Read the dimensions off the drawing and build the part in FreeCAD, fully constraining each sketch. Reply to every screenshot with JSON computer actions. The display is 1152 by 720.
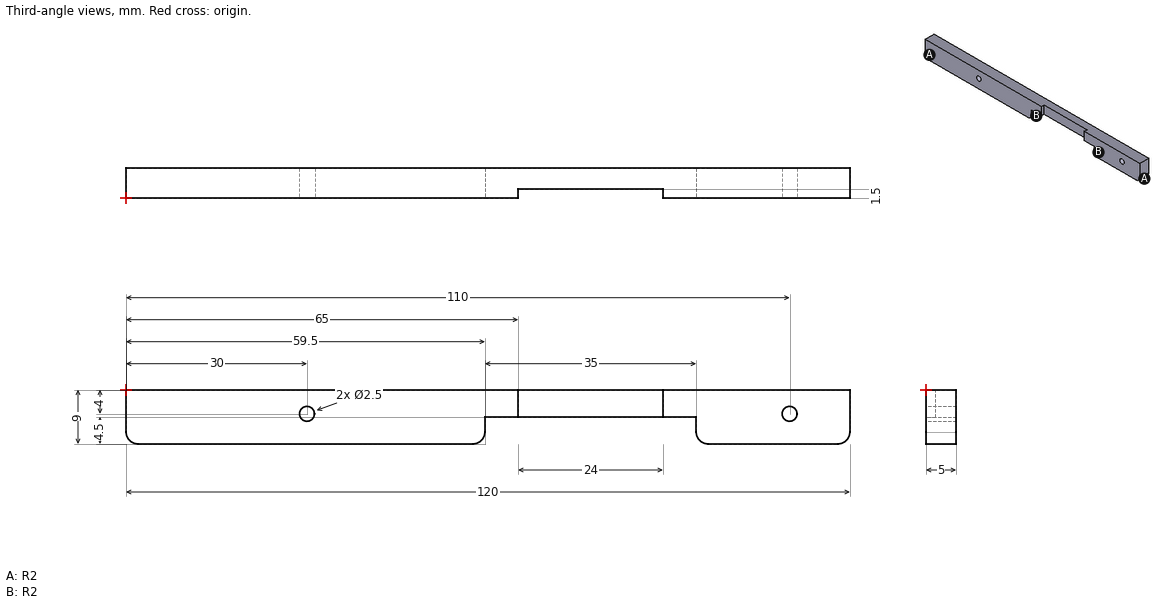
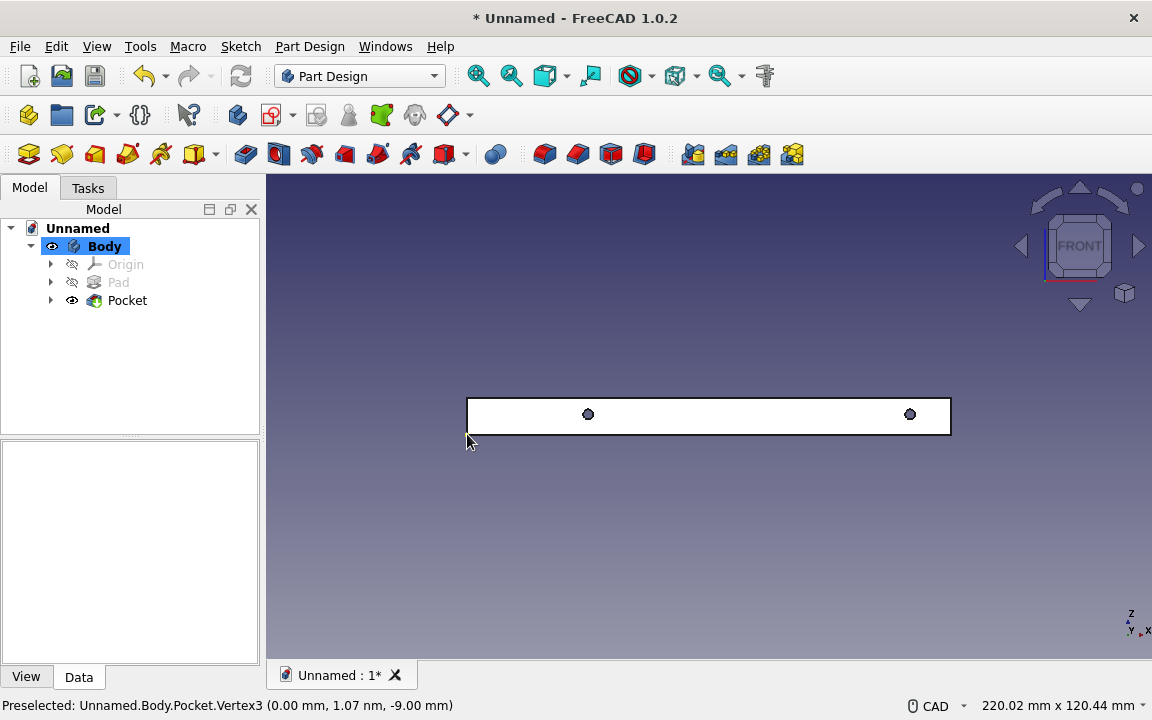
{"action": "key", "text": "3"}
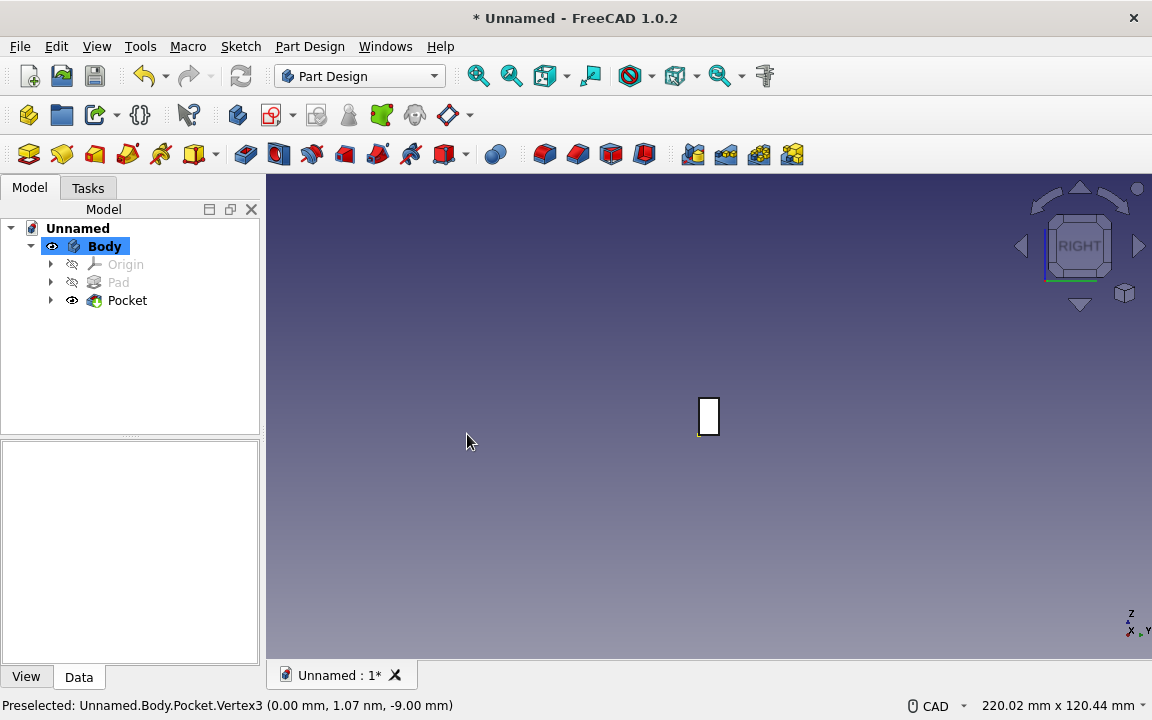
{"action": "key", "text": "v f"}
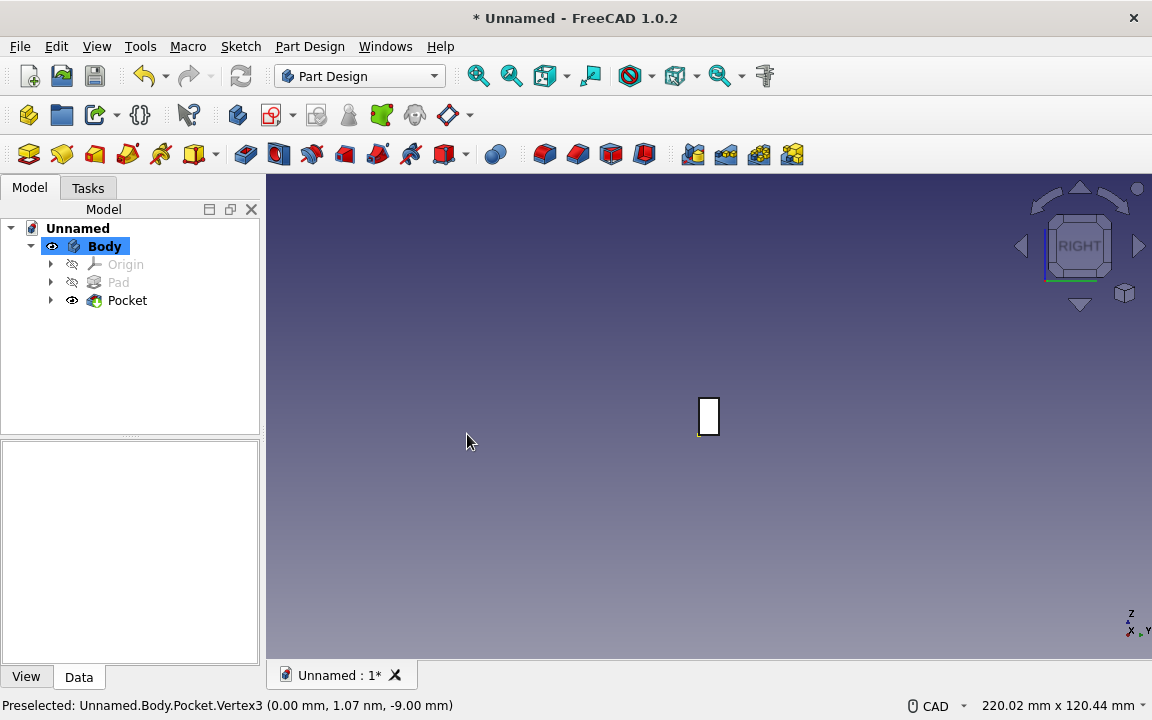
{"action": "left_click", "coordinate": [709, 434]}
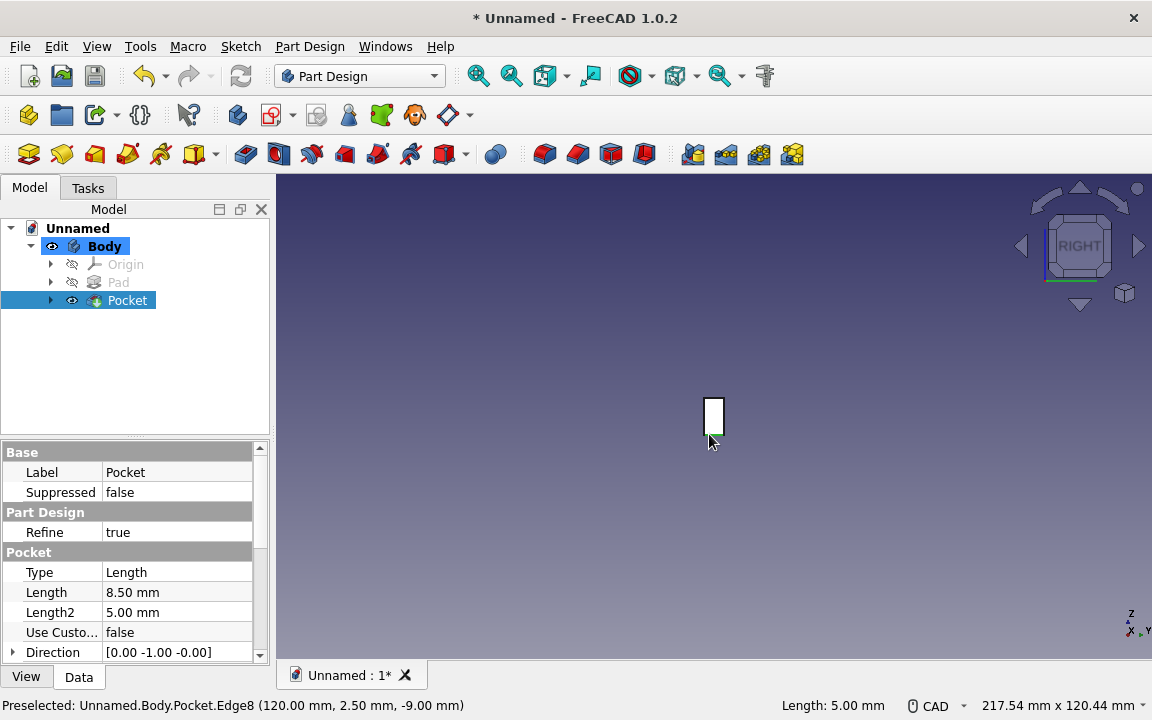
{"action": "scroll", "coordinate": [714, 434], "scroll_direction": "up", "scroll_amount": 4}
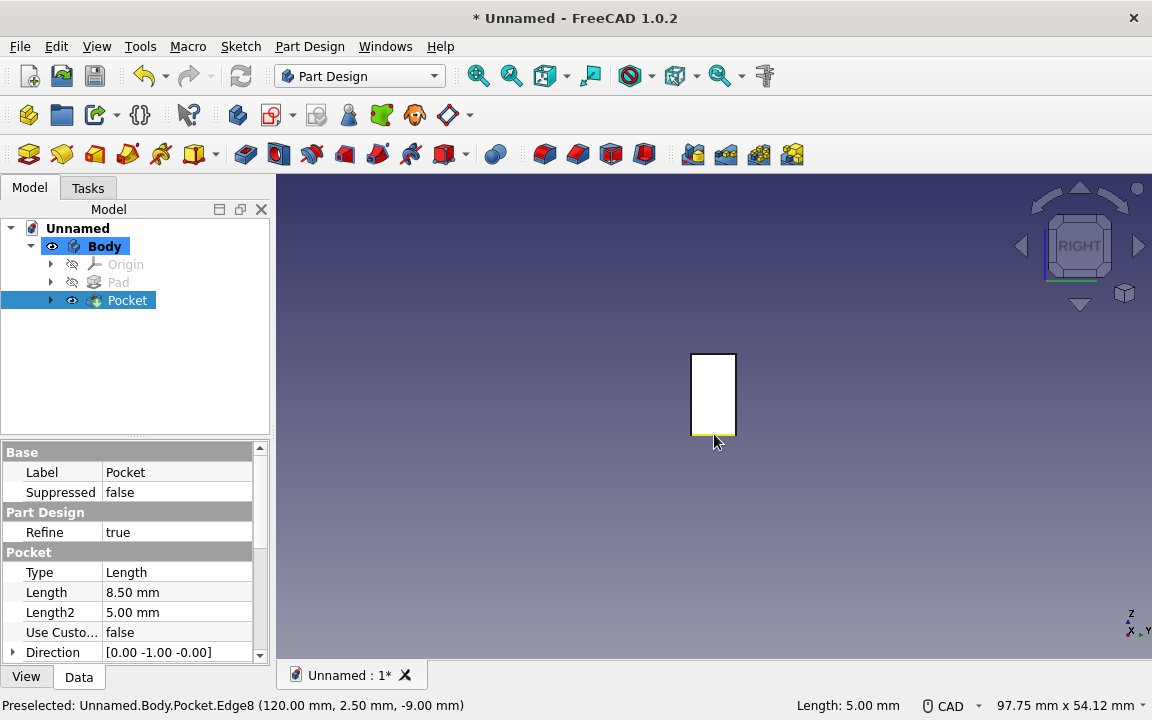
{"action": "key", "text": "v f"}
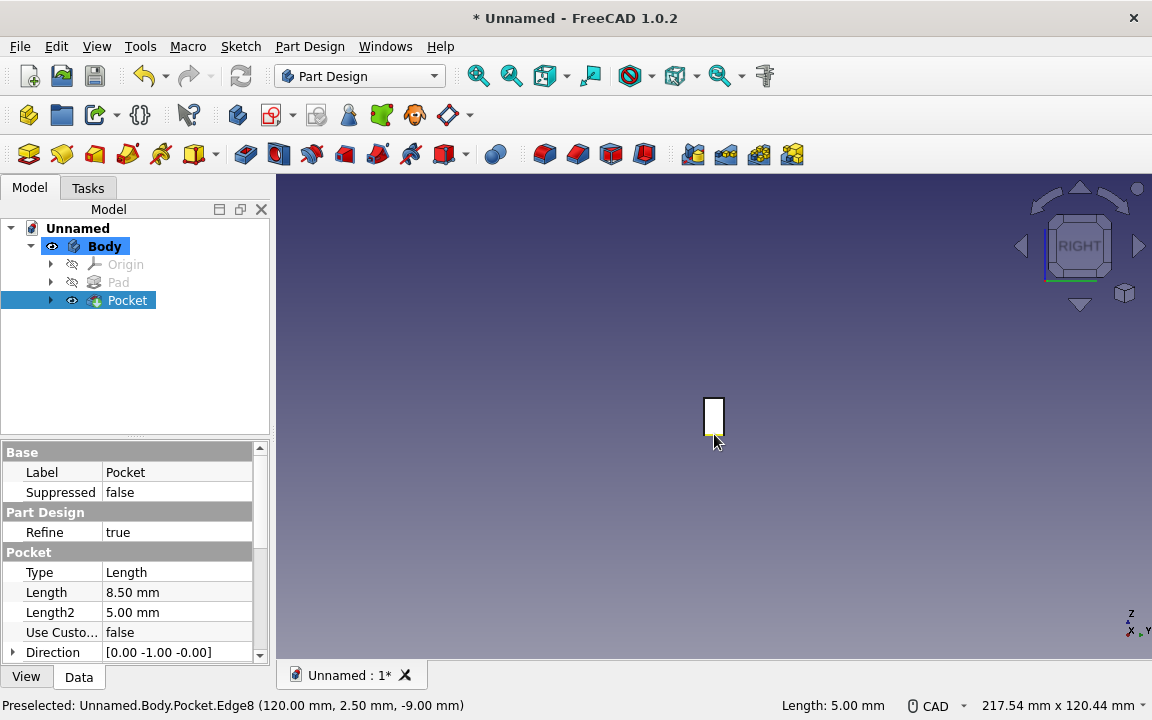
{"action": "key", "text": "5"}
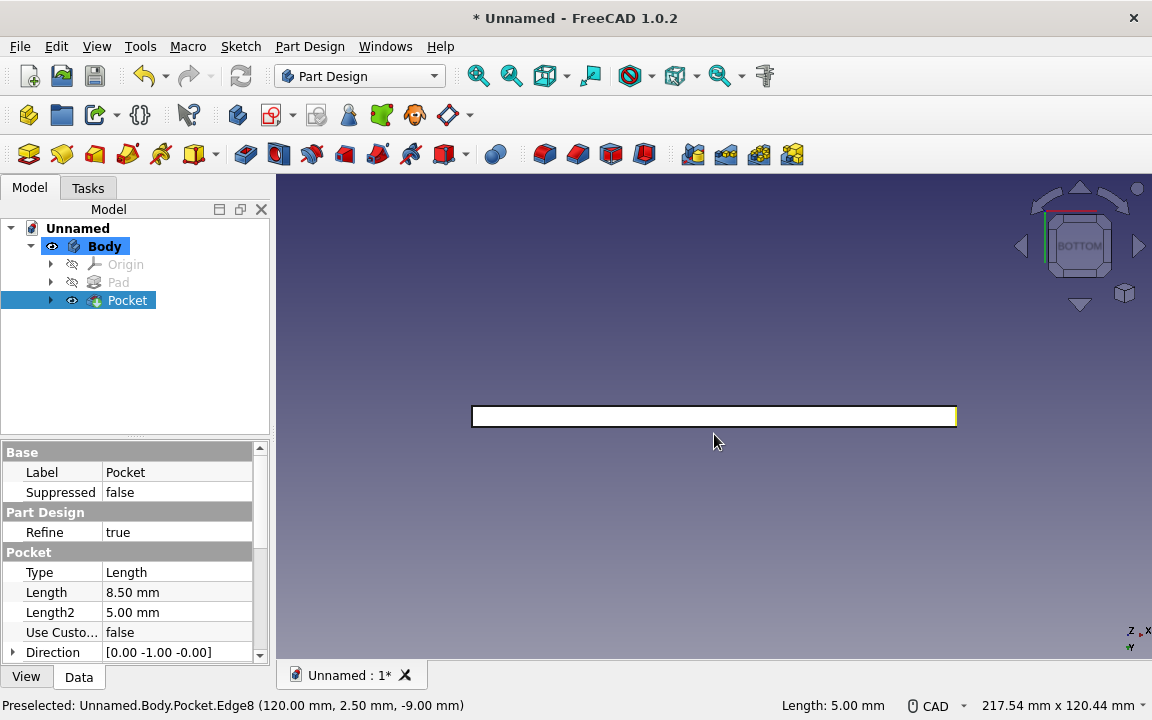
{"action": "left_click", "coordinate": [472, 415], "text": "ctrl"}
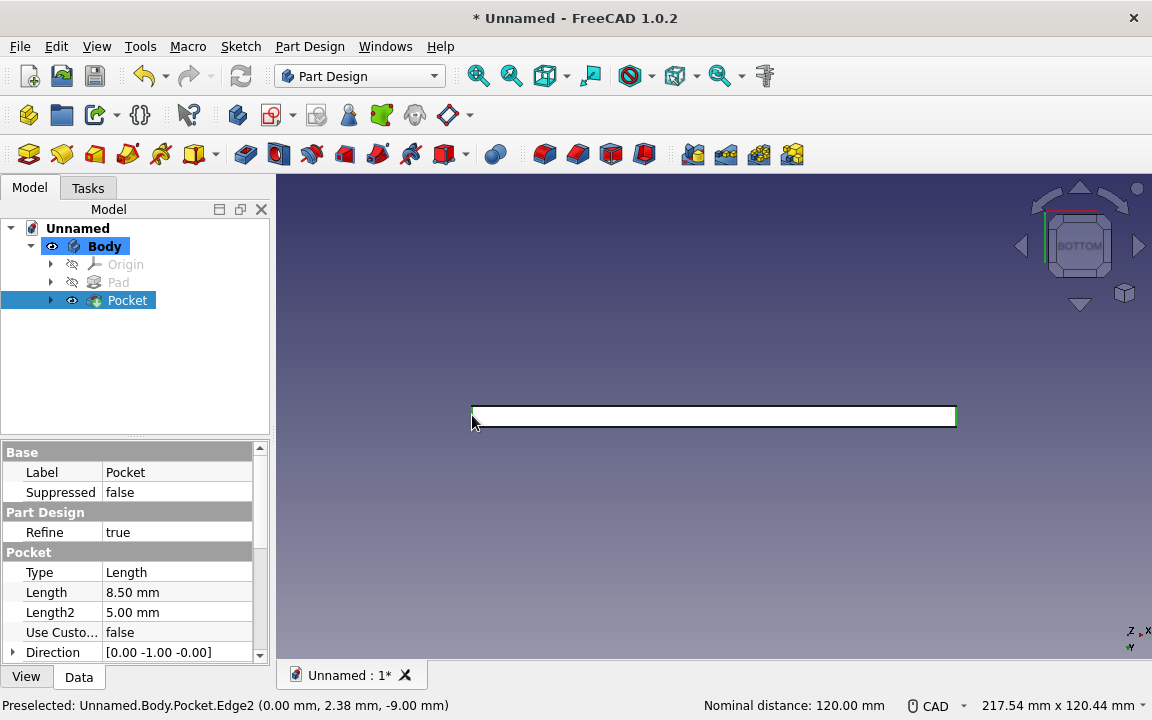
{"action": "left_click", "coordinate": [545, 154]}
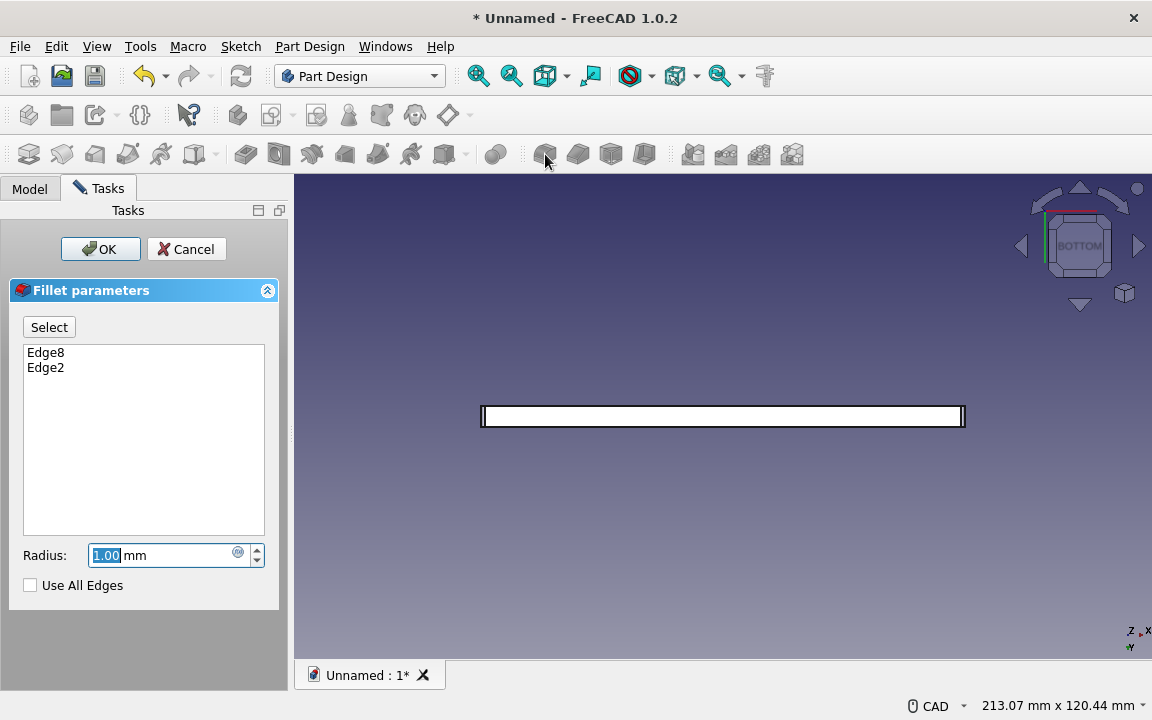
{"action": "type", "text": "2"}
{"action": "key", "text": "Tab"}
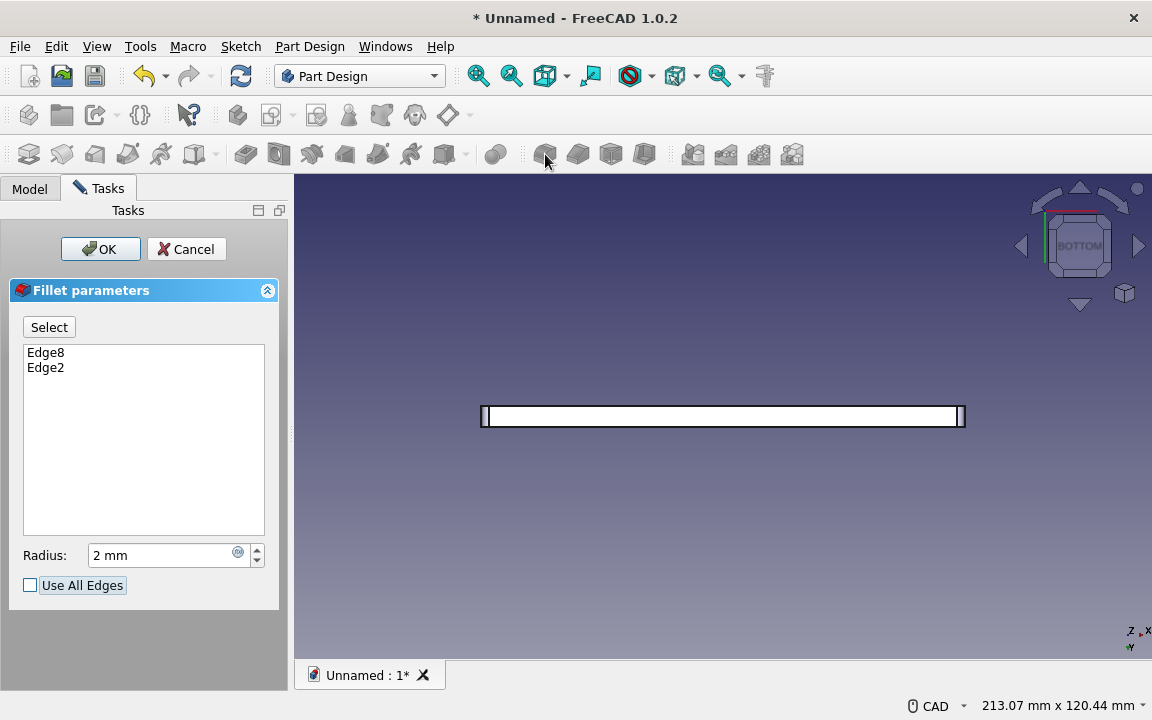
{"action": "left_click", "coordinate": [101, 249]}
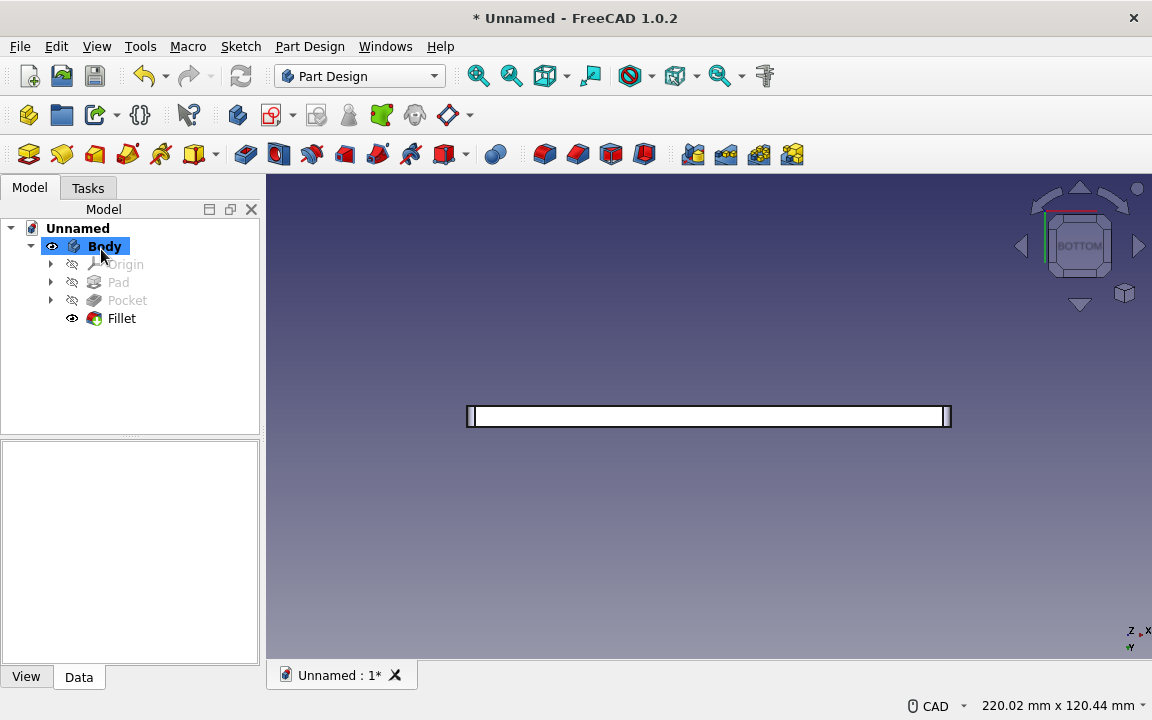
{"action": "key", "text": "4"}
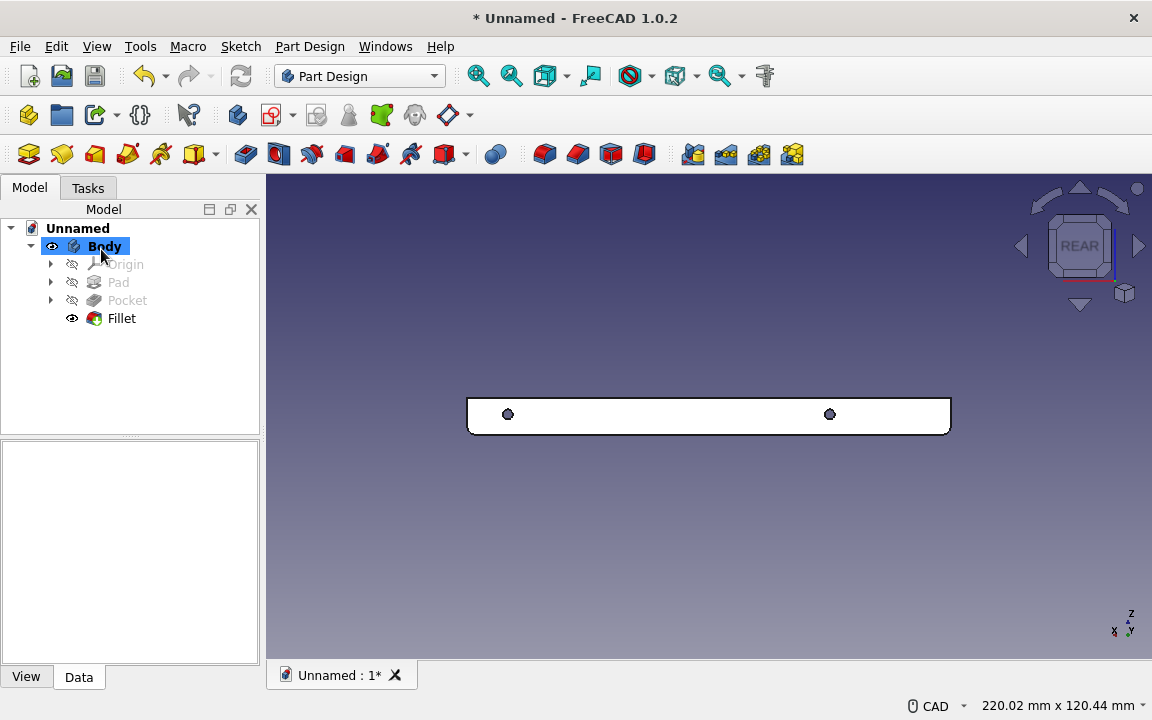
{"action": "left_click", "coordinate": [571, 416]}